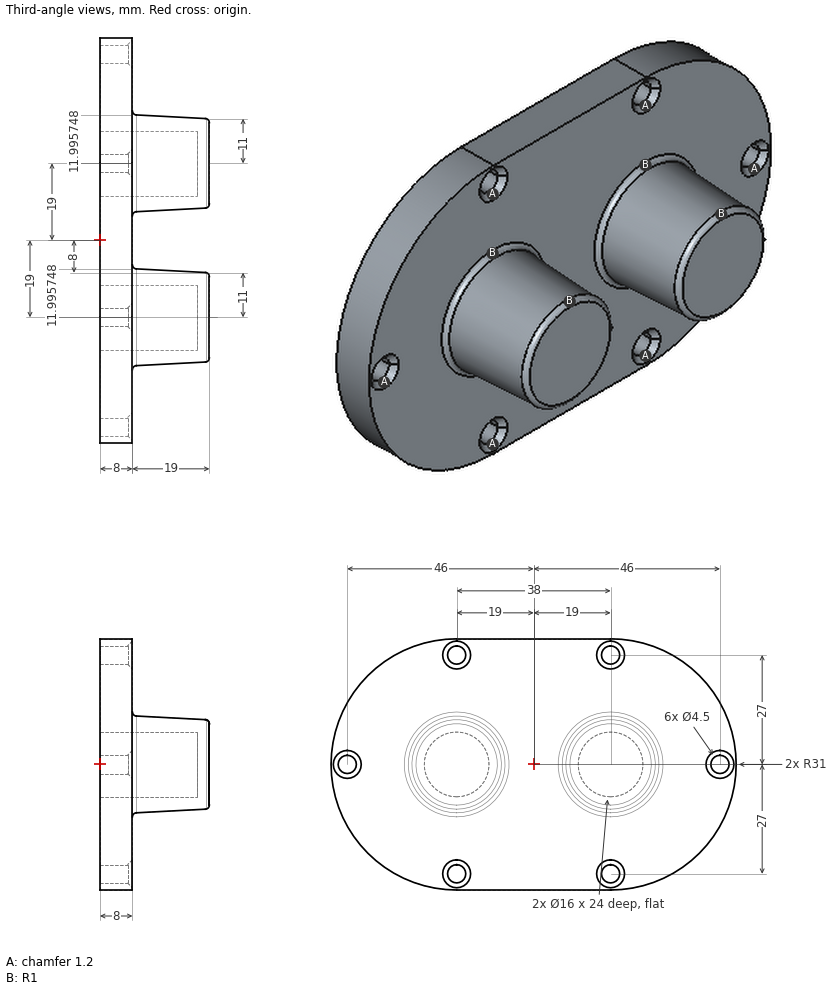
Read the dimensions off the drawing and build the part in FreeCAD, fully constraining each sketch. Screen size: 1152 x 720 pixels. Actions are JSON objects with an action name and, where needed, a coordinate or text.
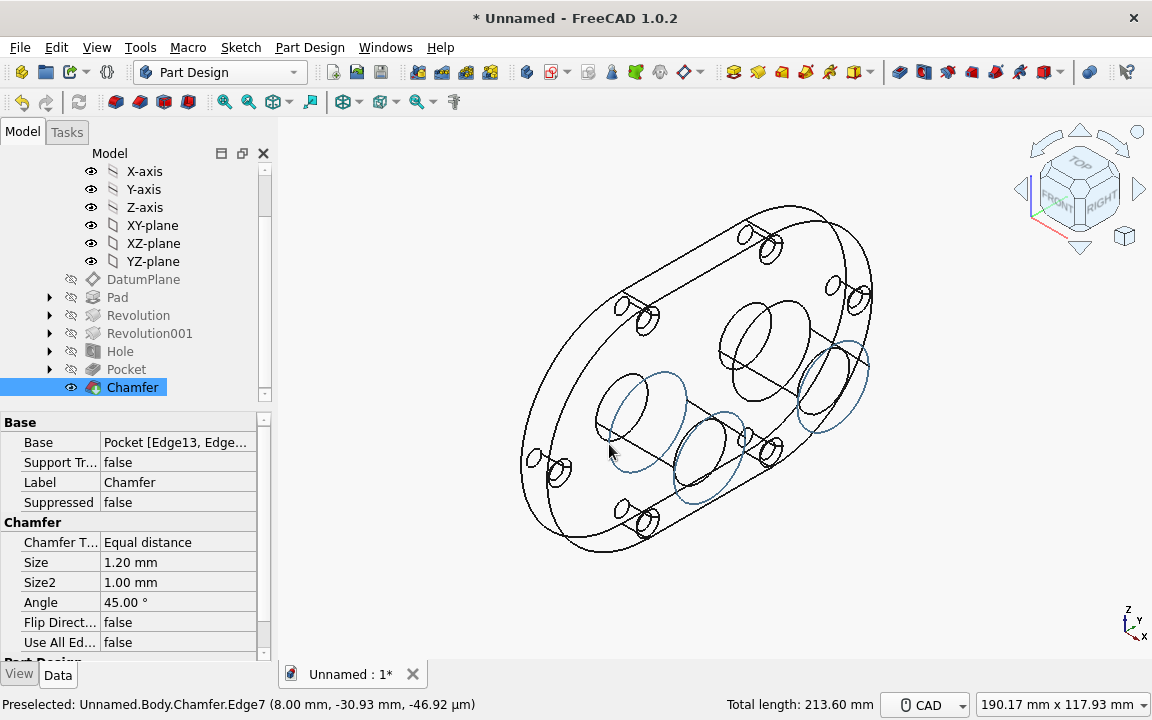
{"action": "left_click", "coordinate": [732, 373], "text": "ctrl"}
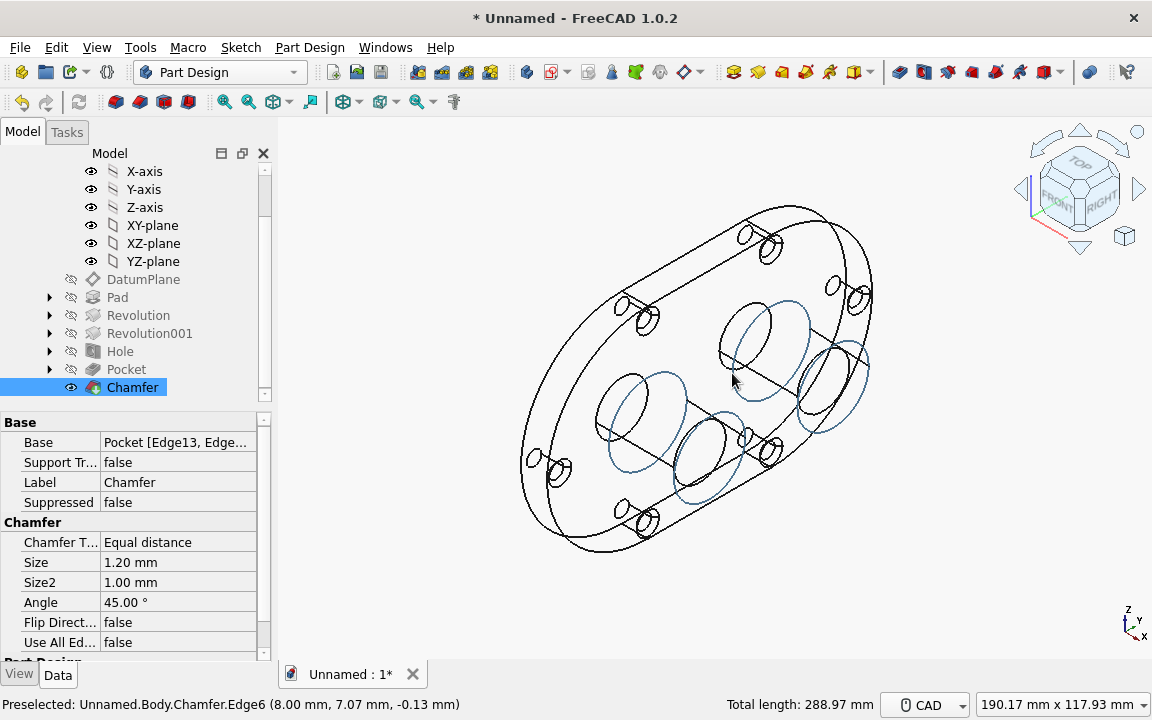
{"action": "key", "text": "v 1"}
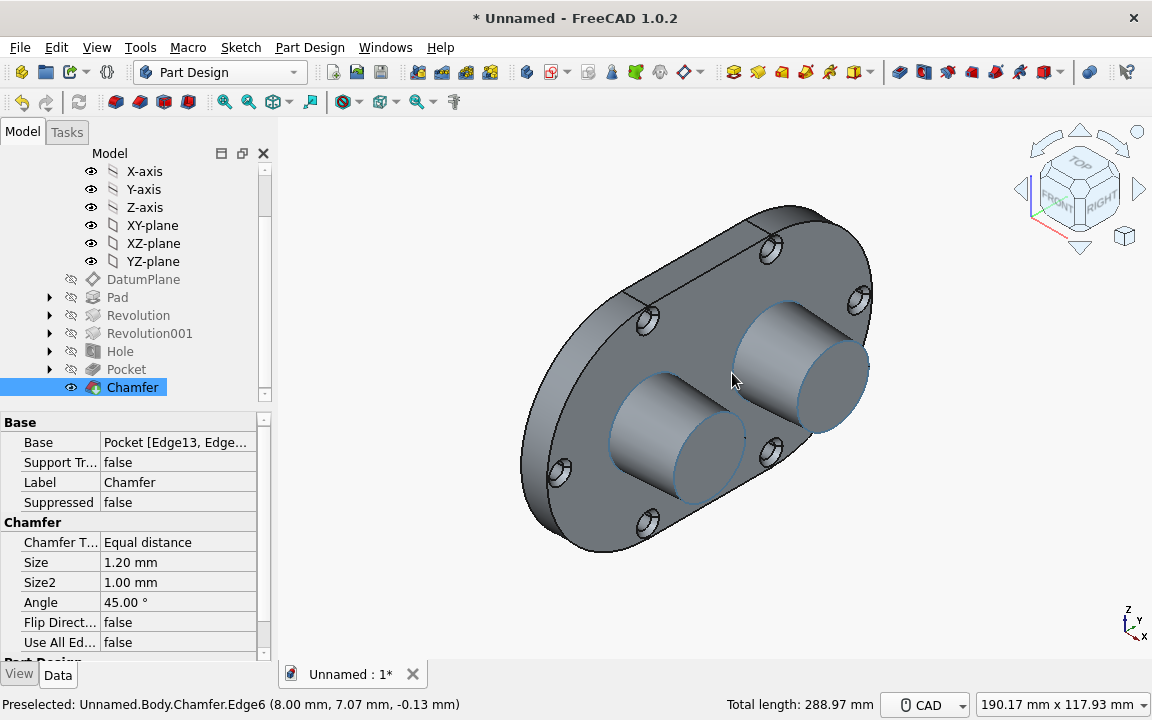
{"action": "left_click", "coordinate": [116, 102]}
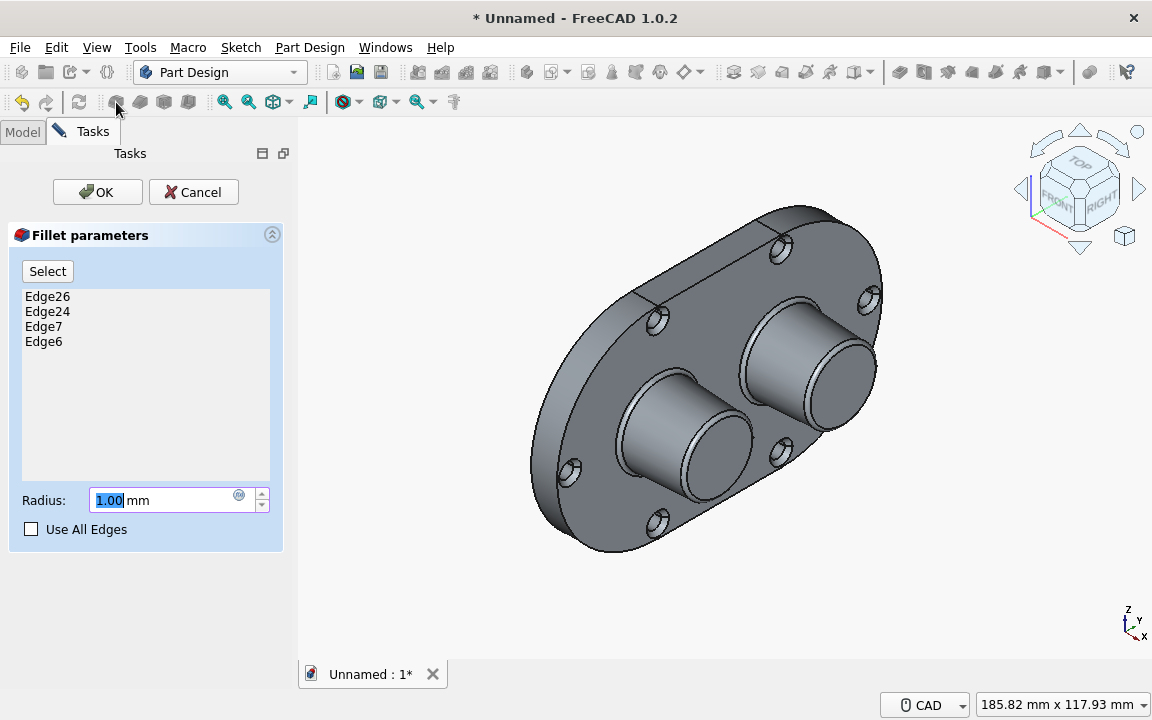
{"action": "type", "text": "1"}
{"action": "key", "text": "Tab"}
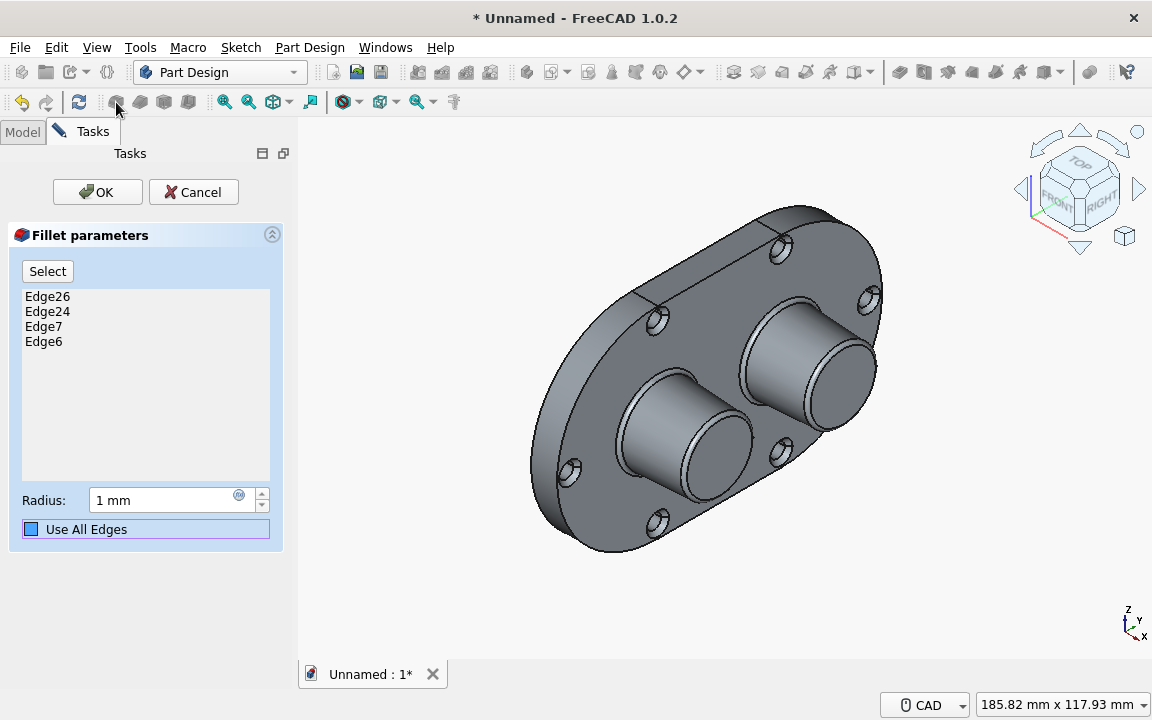
{"action": "left_click", "coordinate": [98, 192]}